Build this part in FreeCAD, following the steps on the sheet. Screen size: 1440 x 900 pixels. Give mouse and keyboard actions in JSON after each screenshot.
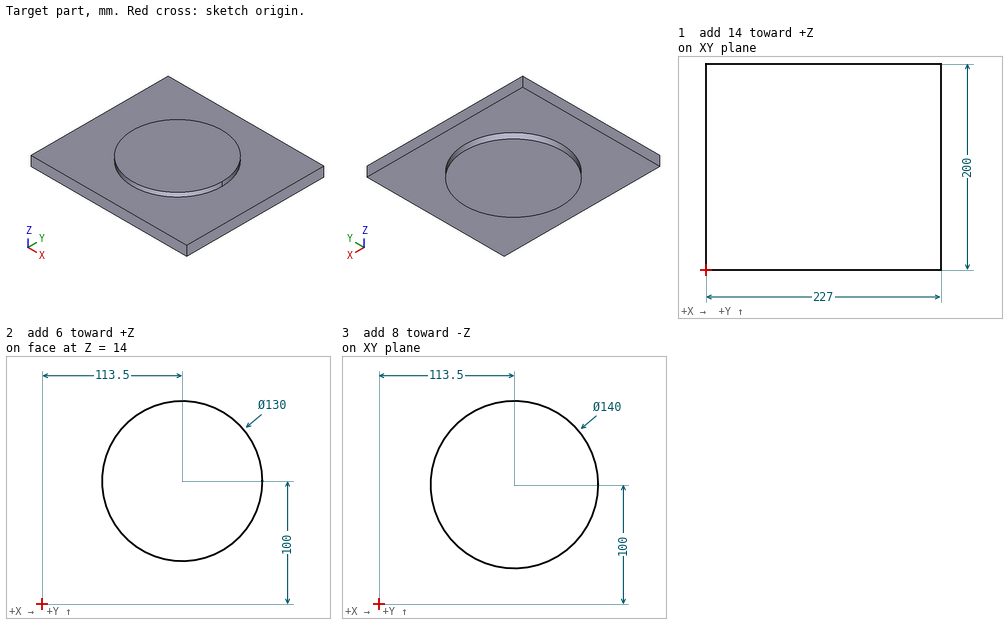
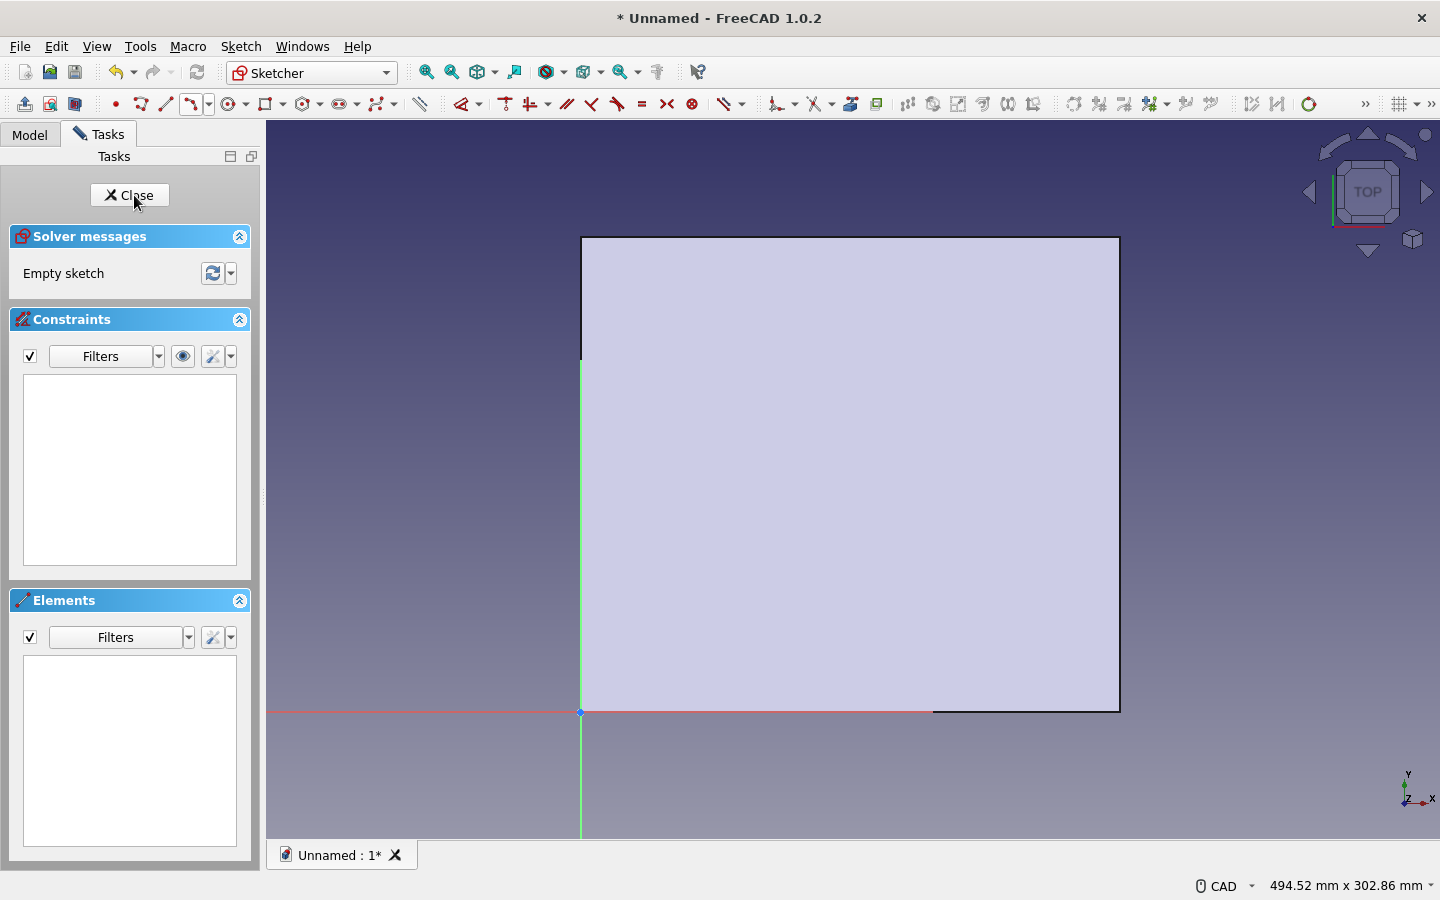
{"action": "left_click", "coordinate": [228, 104]}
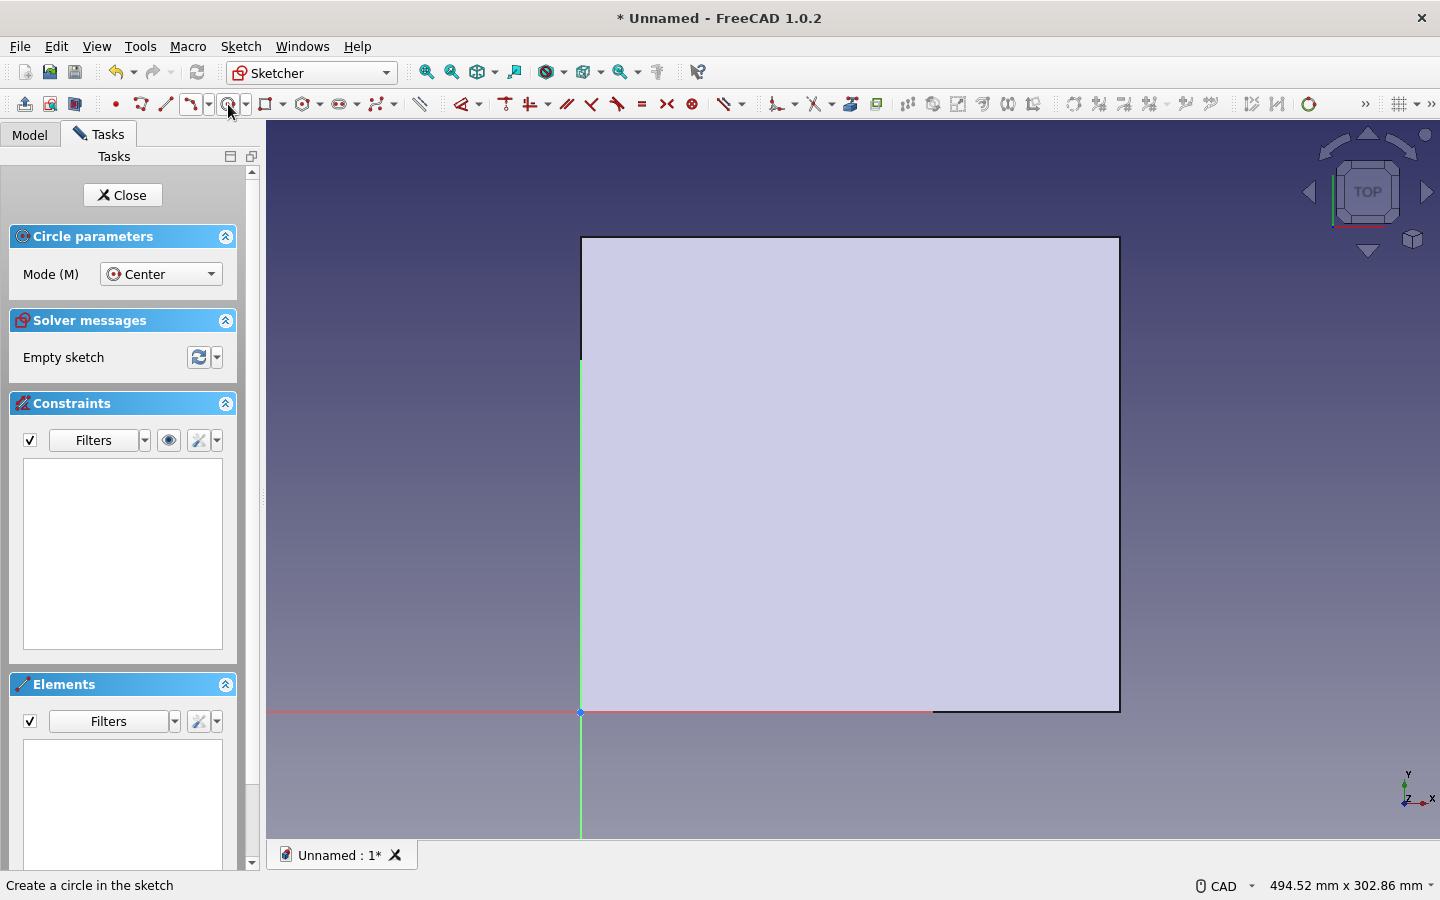
{"action": "left_click", "coordinate": [850, 475]}
{"action": "mouse_move", "coordinate": [968, 357]}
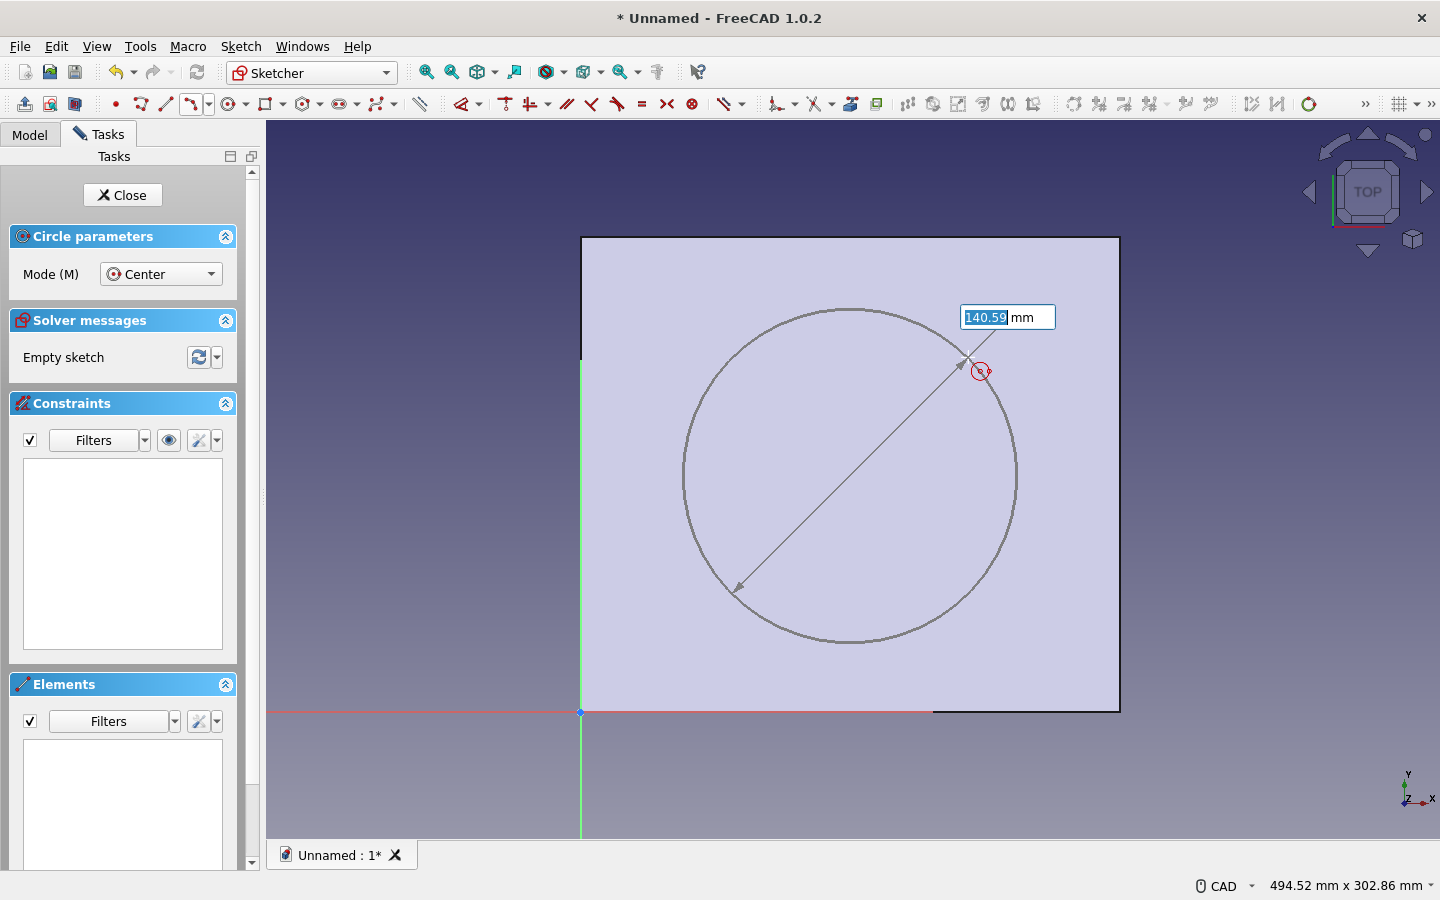
{"action": "type", "text": "140"}
{"action": "key", "text": "Return"}
{"action": "key", "text": "Escape"}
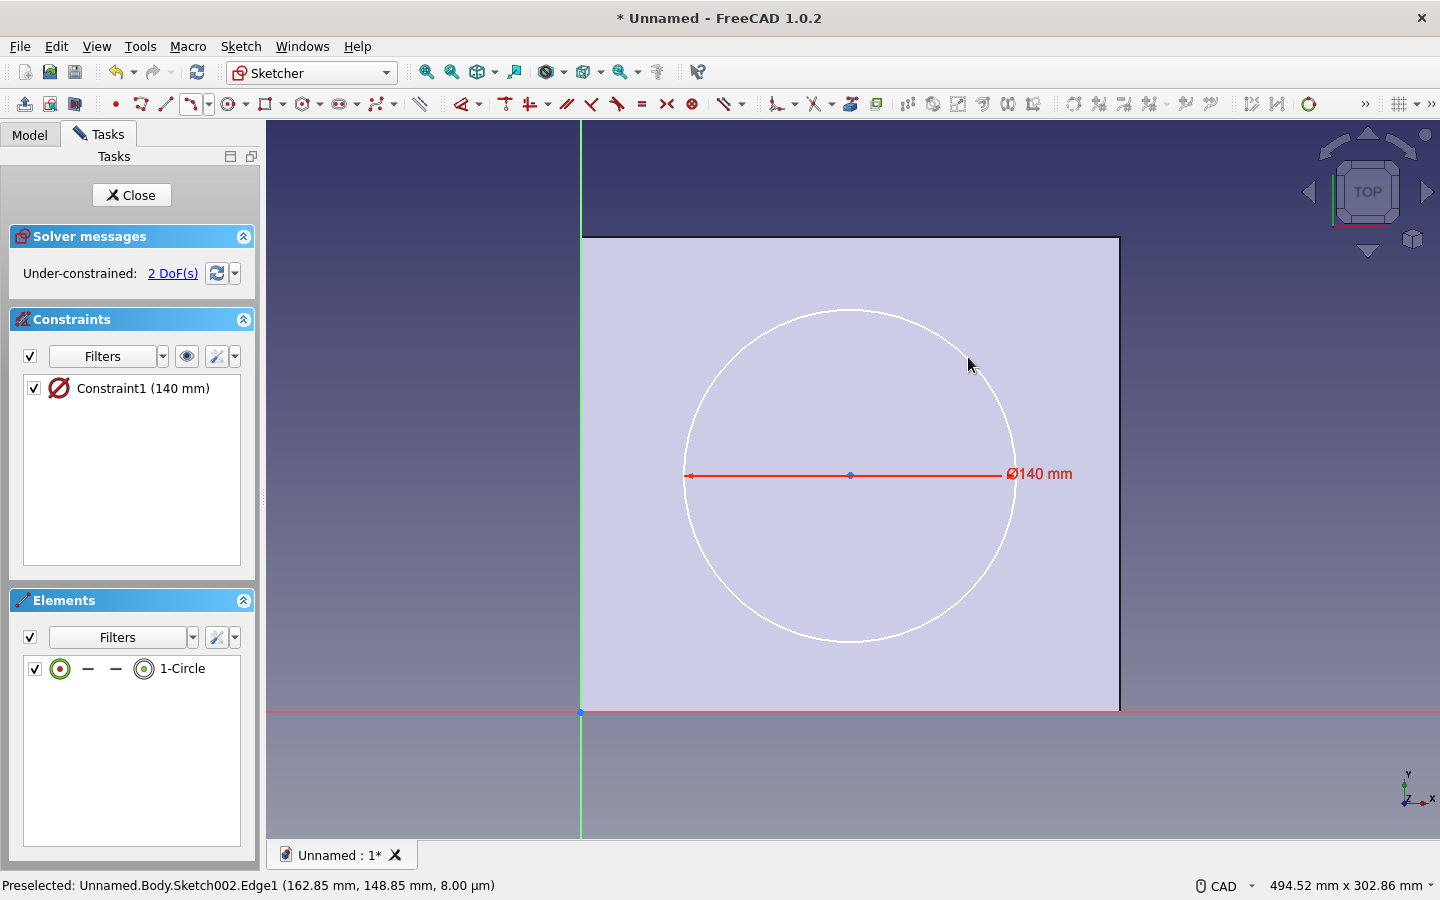
{"action": "left_click", "coordinate": [850, 476]}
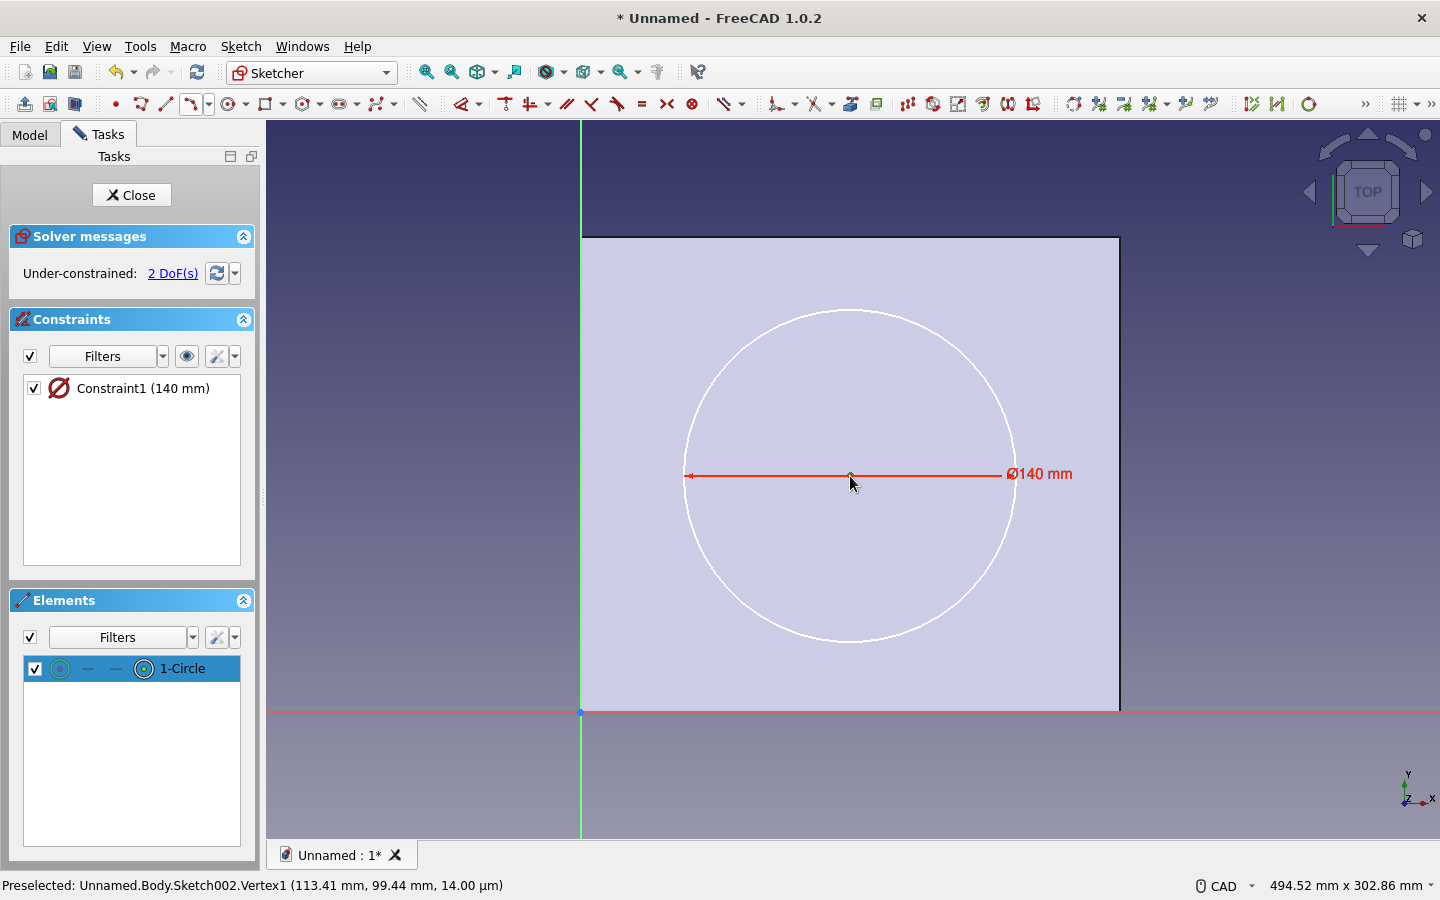
{"action": "key", "text": "i"}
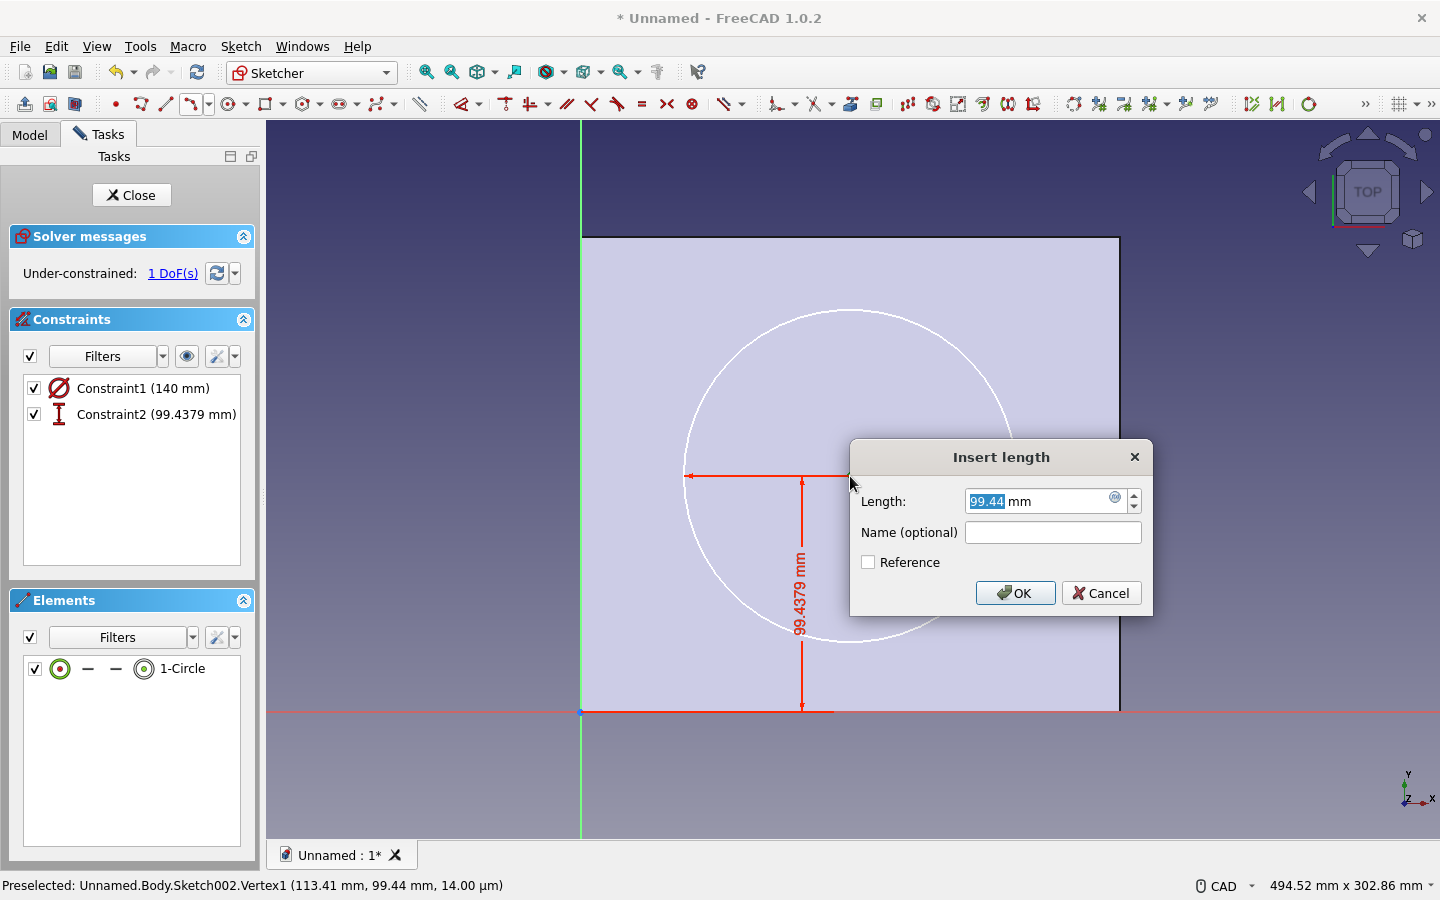
{"action": "type", "text": "100"}
{"action": "key", "text": "Return"}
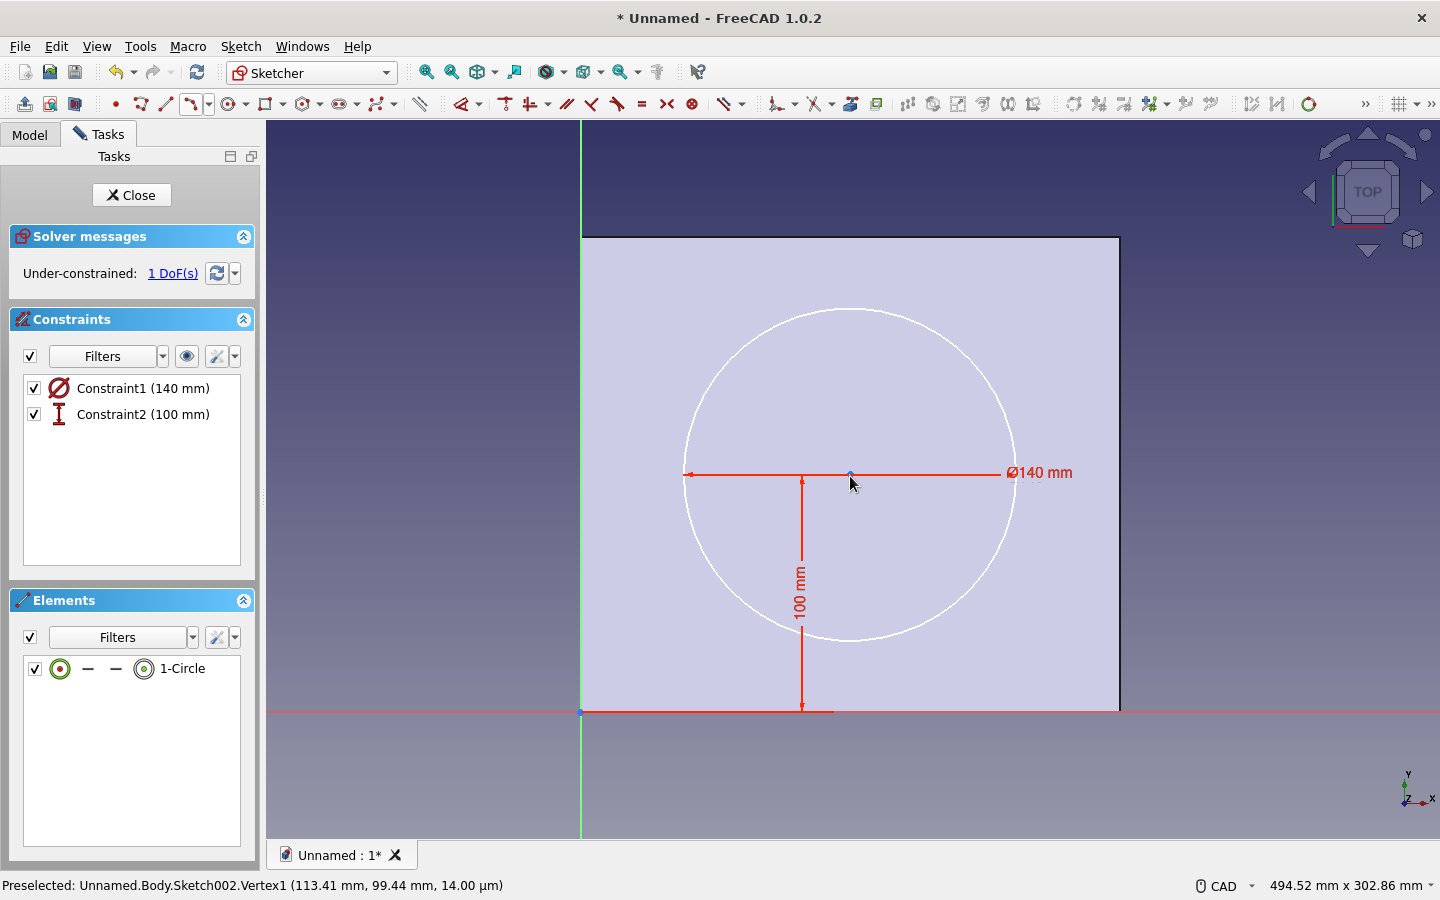
{"action": "left_click", "coordinate": [850, 475]}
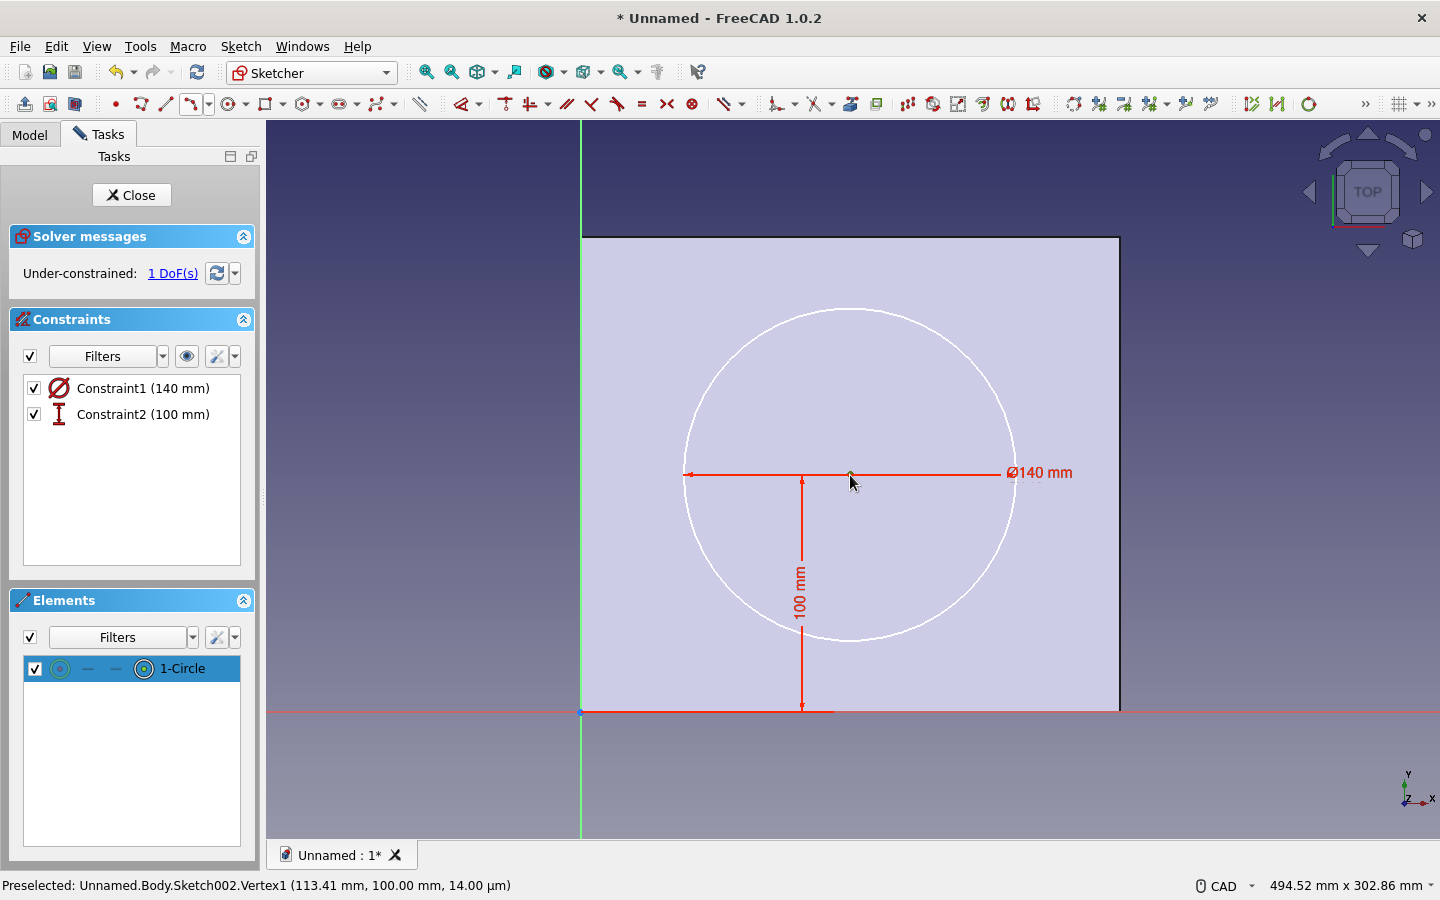
{"action": "key", "text": "l"}